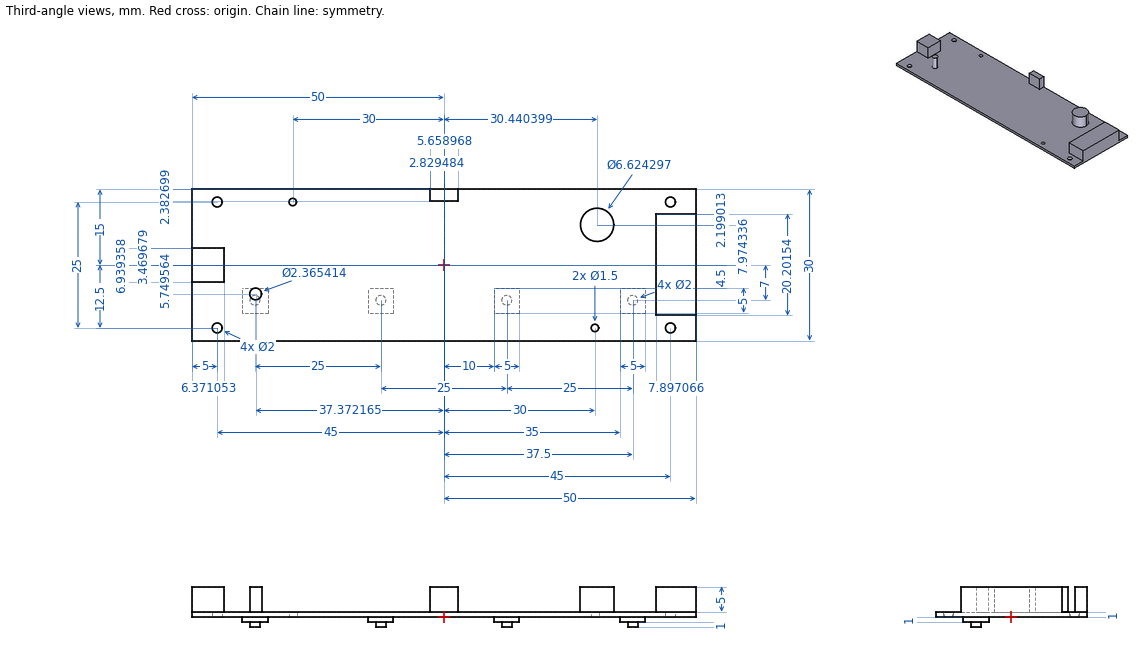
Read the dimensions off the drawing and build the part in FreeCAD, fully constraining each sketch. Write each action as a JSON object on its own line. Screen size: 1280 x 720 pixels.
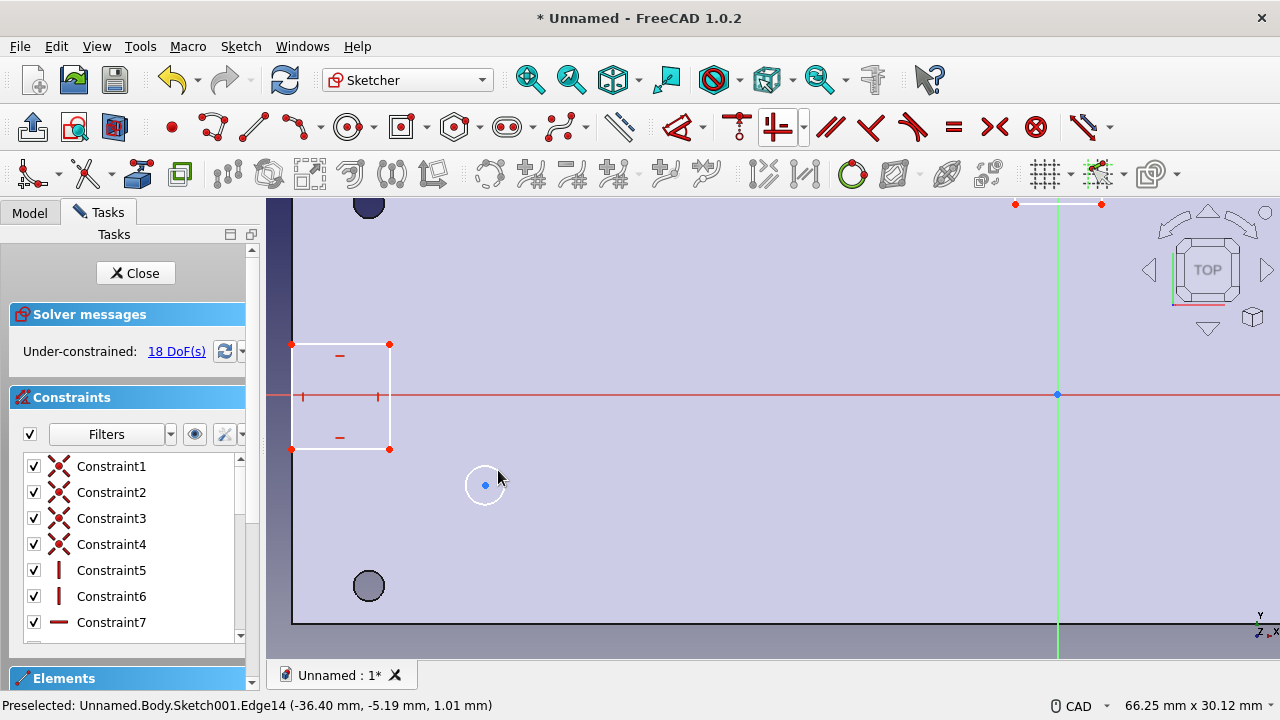
{"action": "key", "text": "d"}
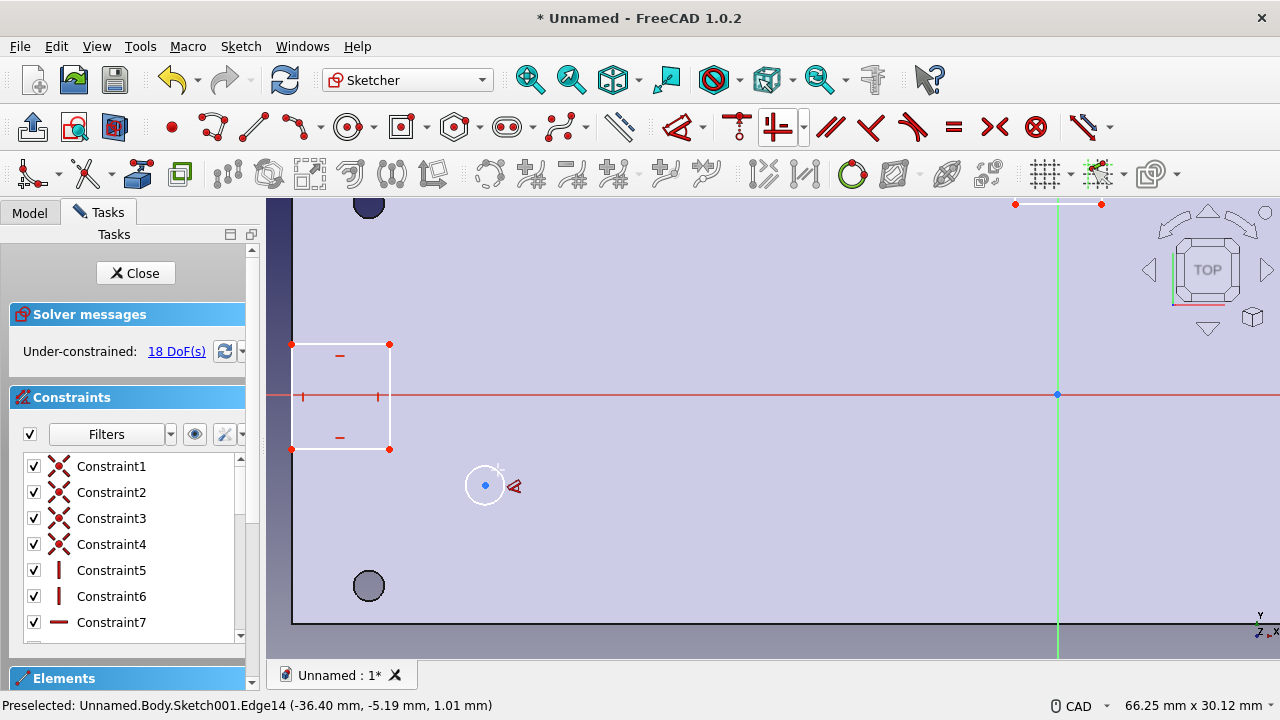
{"action": "scroll", "coordinate": [499, 470], "scroll_direction": "down", "scroll_amount": 5}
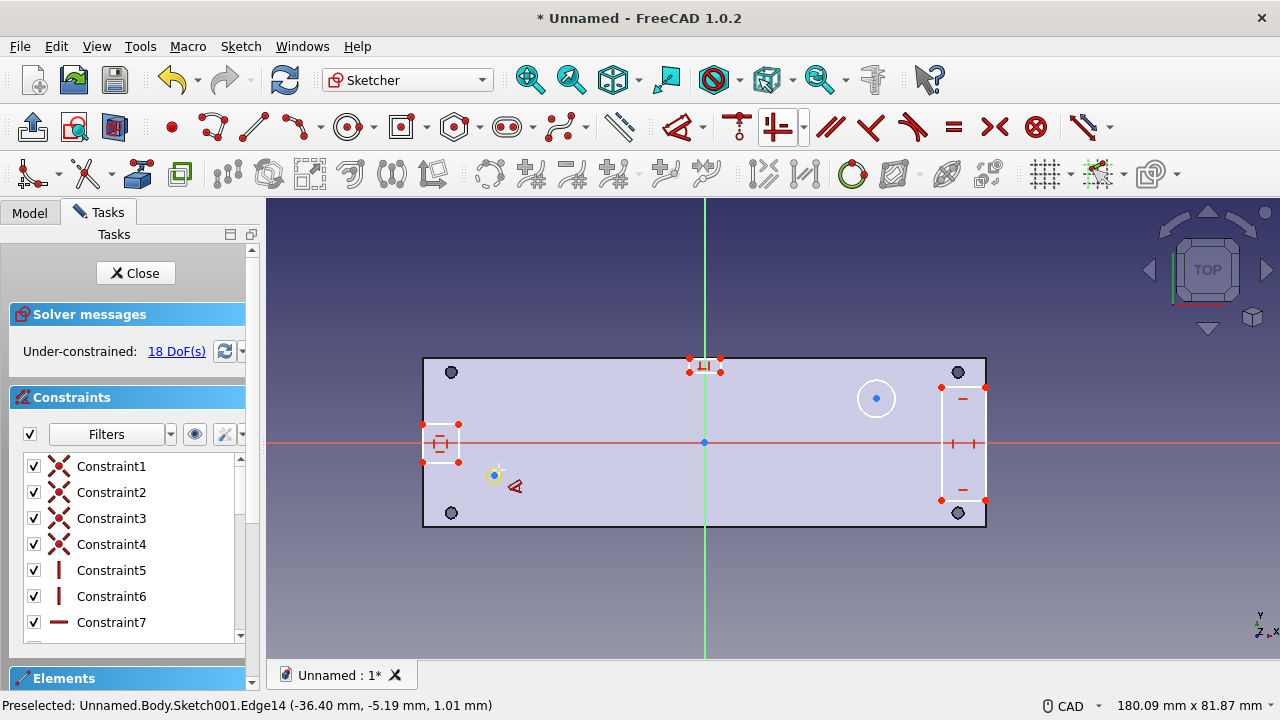
{"action": "left_click", "coordinate": [890, 386]}
{"action": "left_click", "coordinate": [913, 364]}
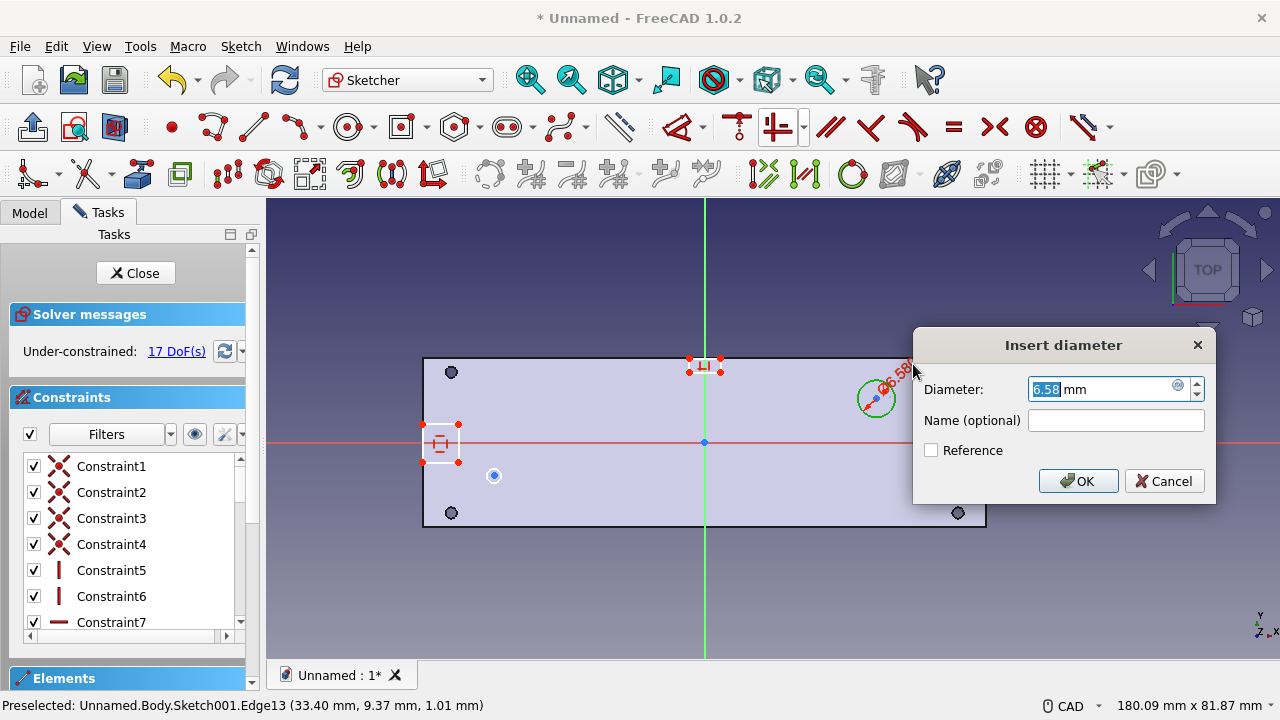
{"action": "type", "text": "6.624297"}
{"action": "key", "text": "Return"}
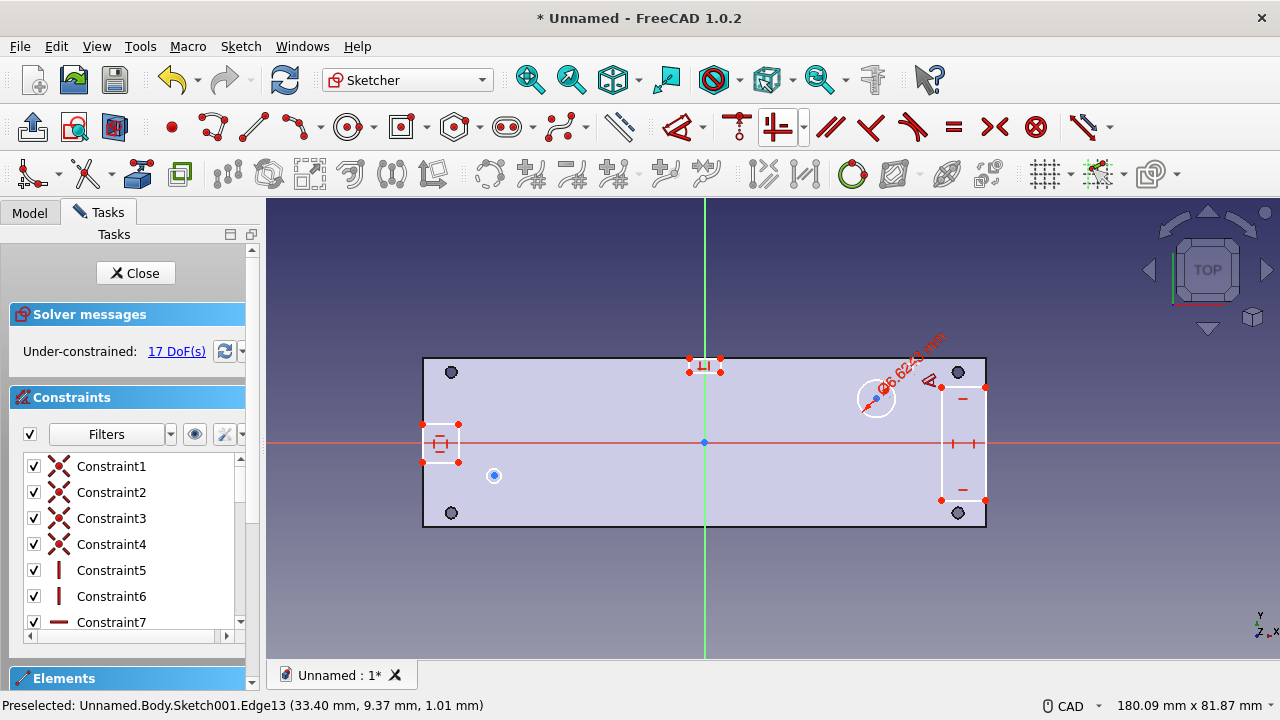
{"action": "scroll", "coordinate": [487, 476], "scroll_direction": "up", "scroll_amount": 6}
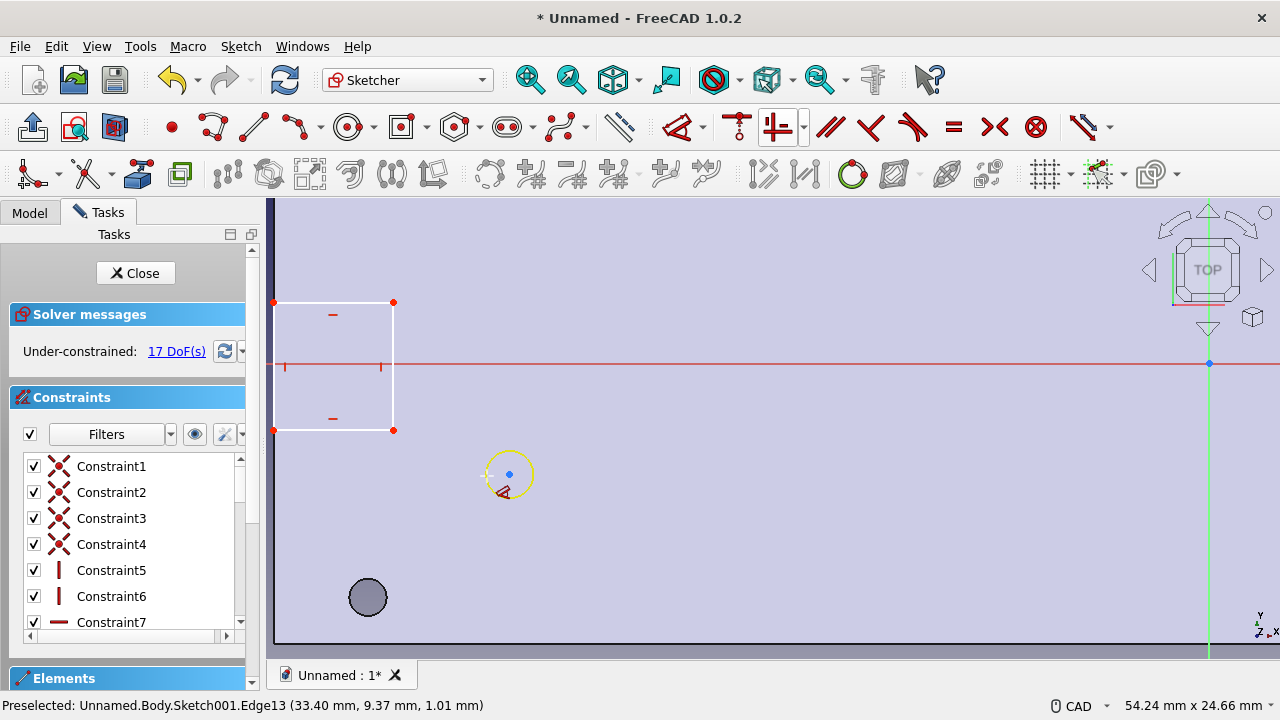
{"action": "left_click", "coordinate": [486, 474]}
{"action": "left_click", "coordinate": [454, 473]}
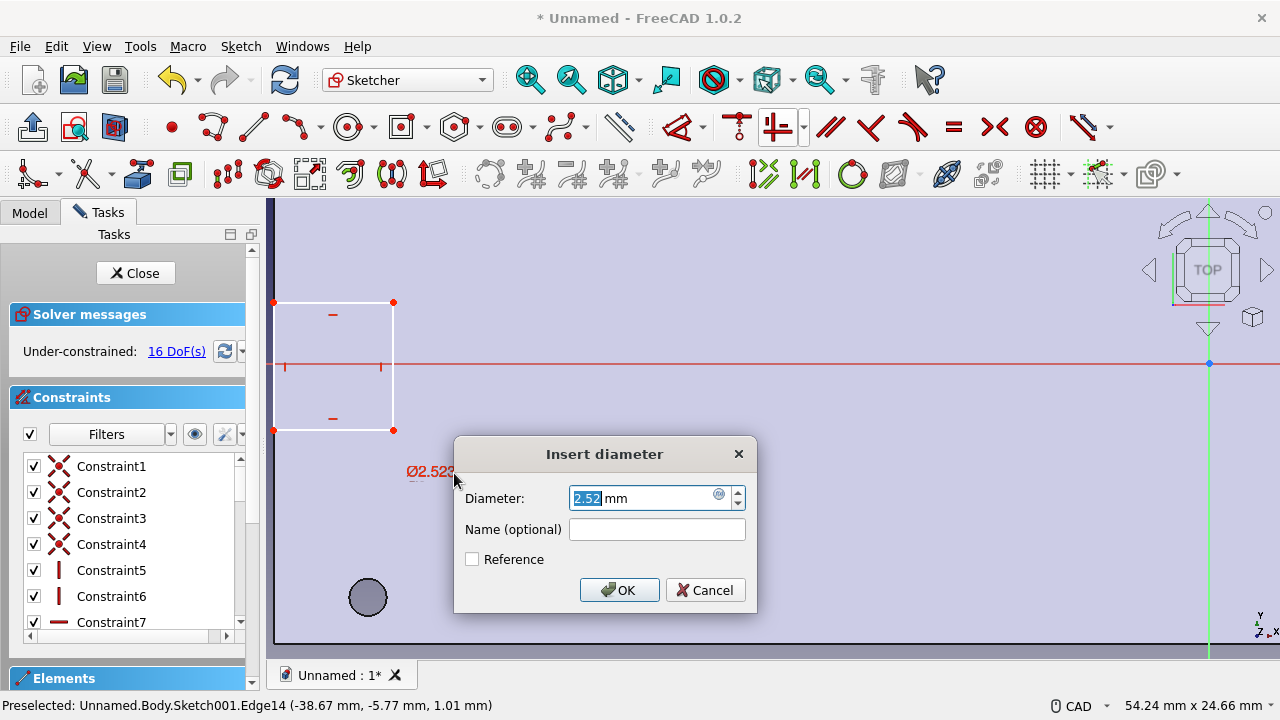
{"action": "type", "text": "2.365414"}
{"action": "key", "text": "Return"}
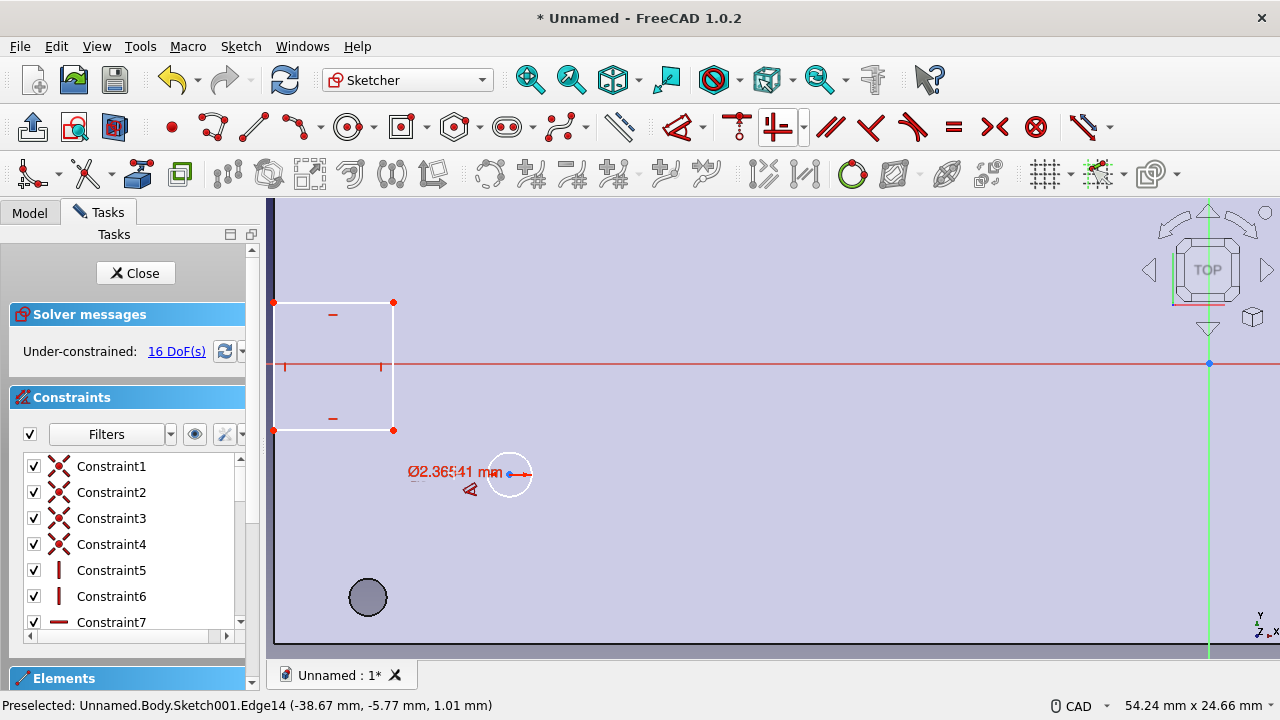
{"action": "scroll", "coordinate": [487, 476], "scroll_direction": "down", "scroll_amount": 6}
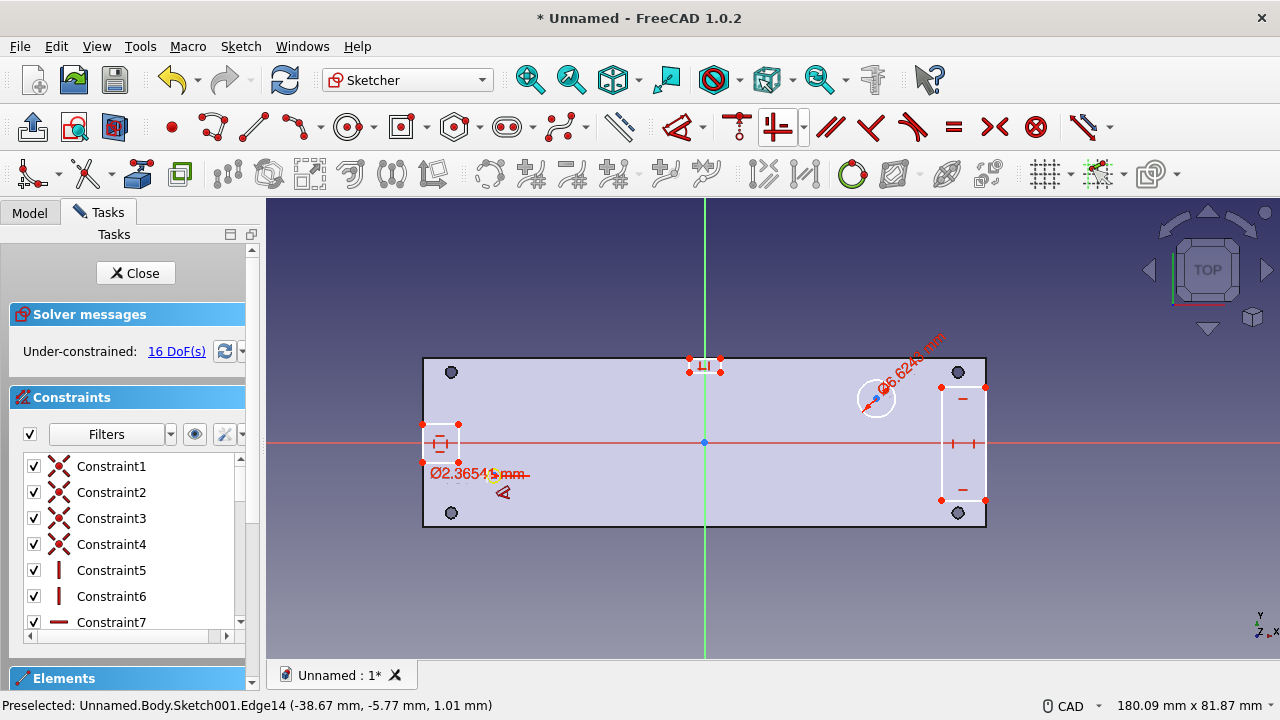
{"action": "left_click", "coordinate": [986, 501]}
{"action": "left_click", "coordinate": [845, 535]}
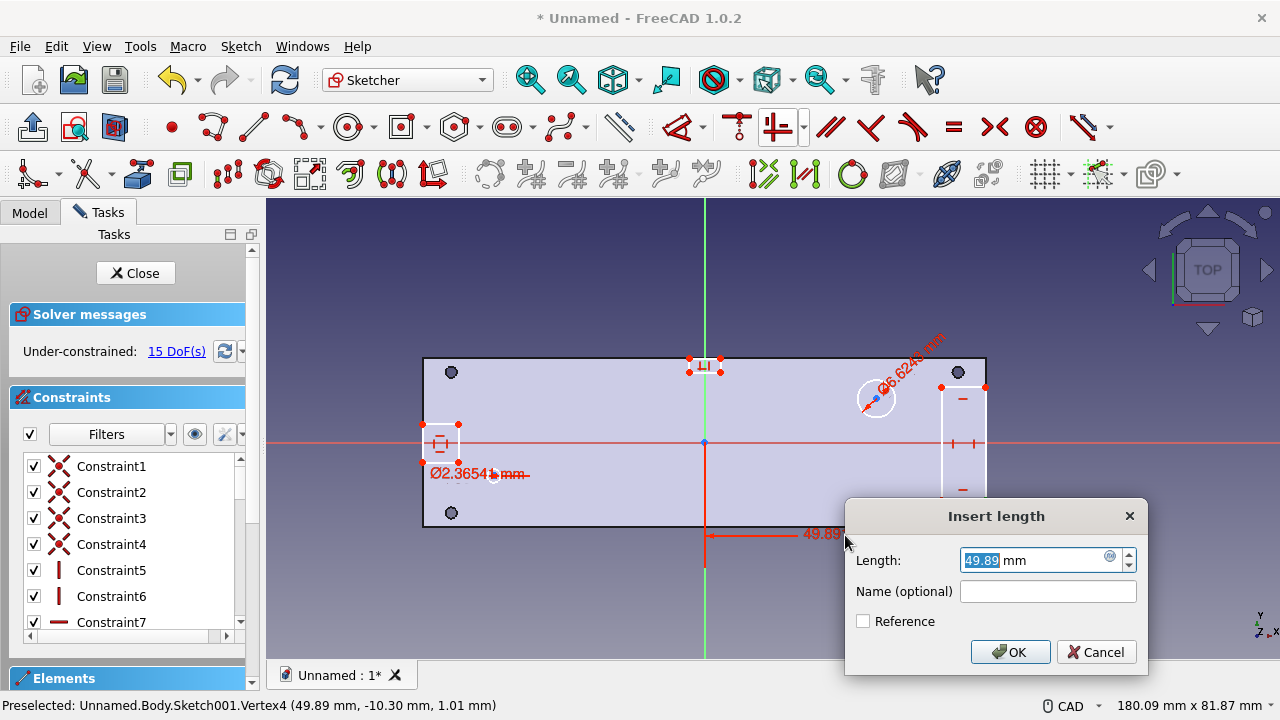
{"action": "type", "text": "50"}
{"action": "key", "text": "Return"}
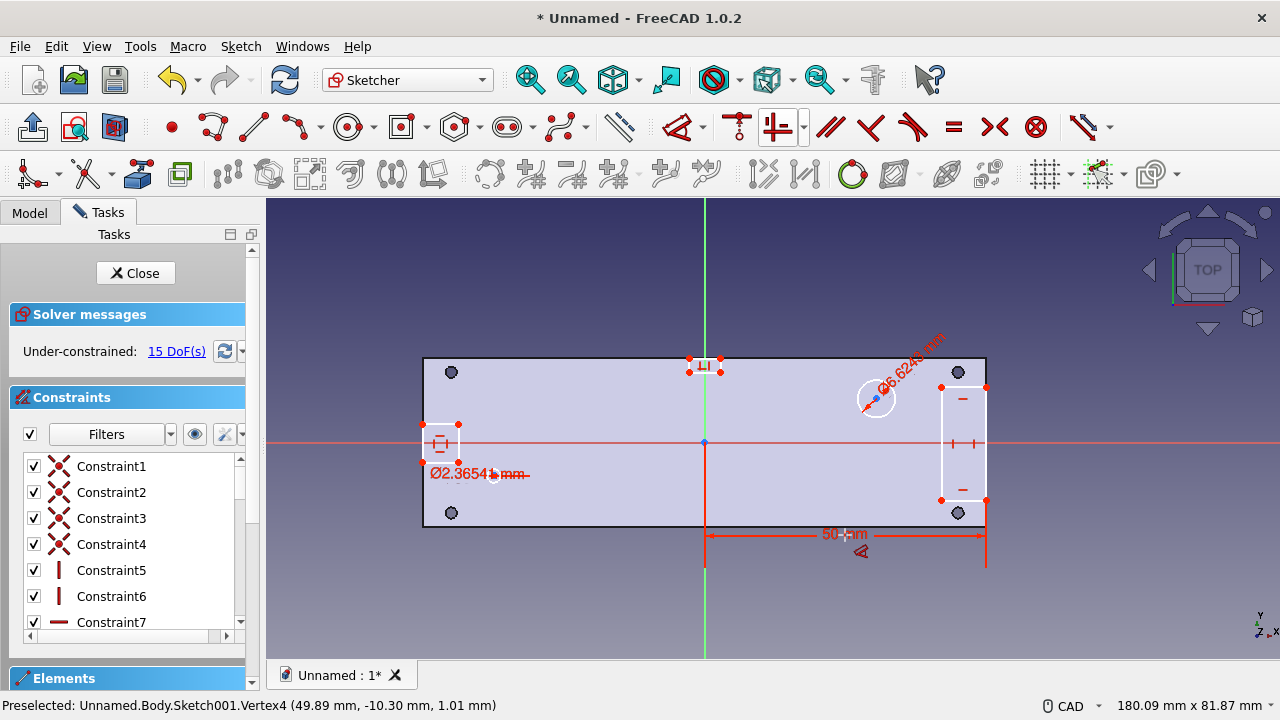
{"action": "left_click", "coordinate": [689, 359]}
{"action": "left_click", "coordinate": [655, 401]}